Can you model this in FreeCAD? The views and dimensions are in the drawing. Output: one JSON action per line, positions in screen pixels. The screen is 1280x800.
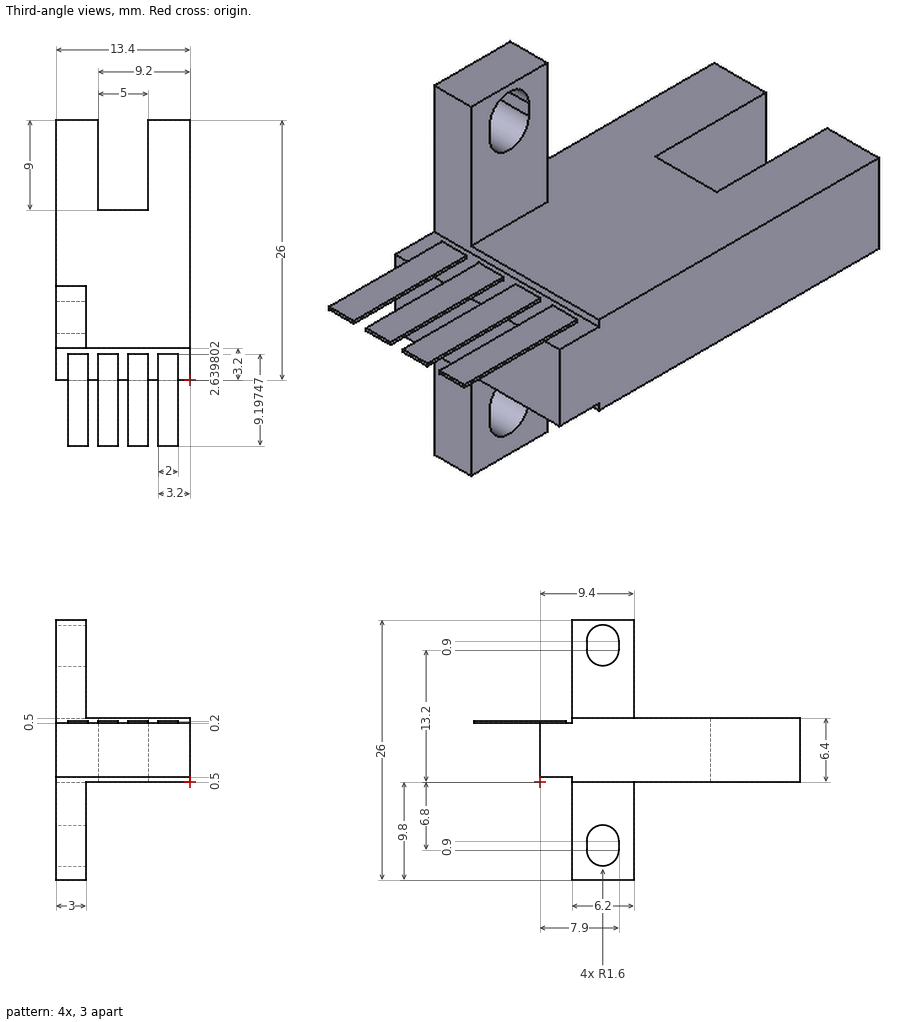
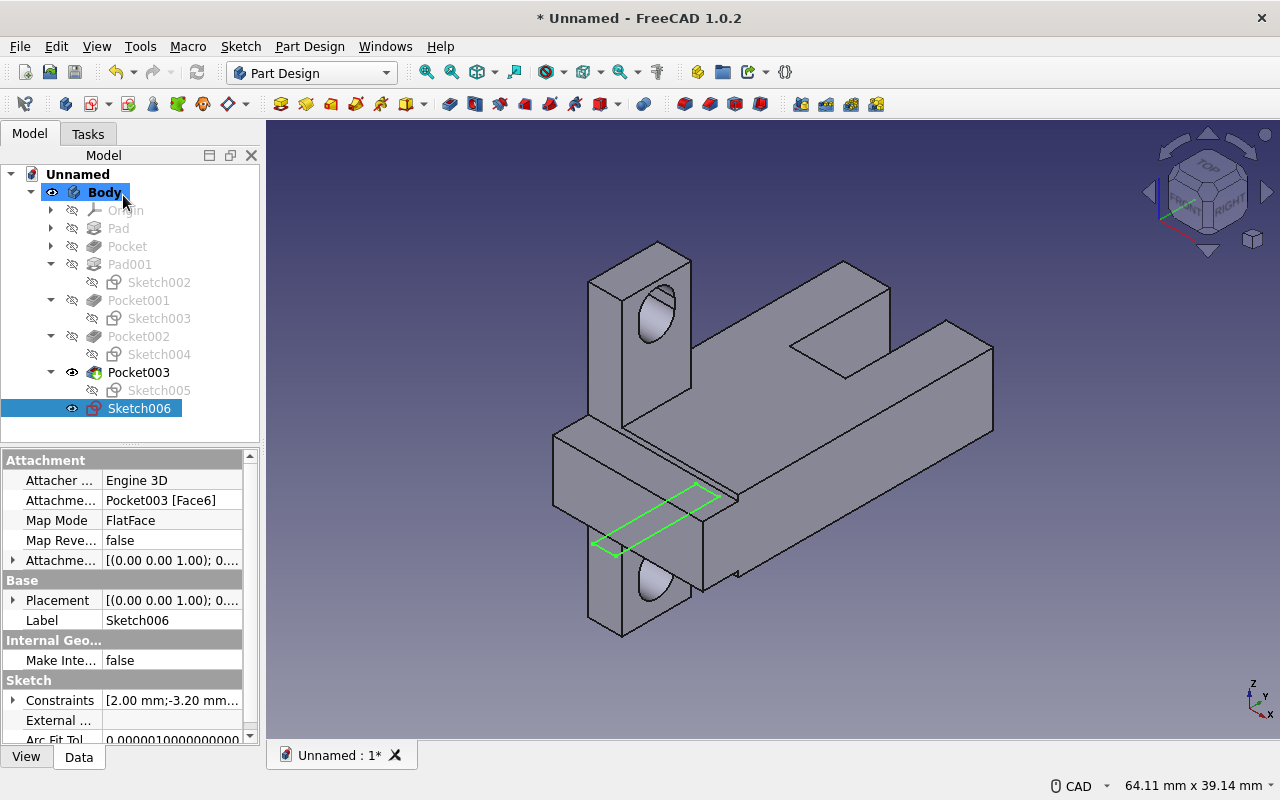
{"action": "left_click", "coordinate": [281, 104]}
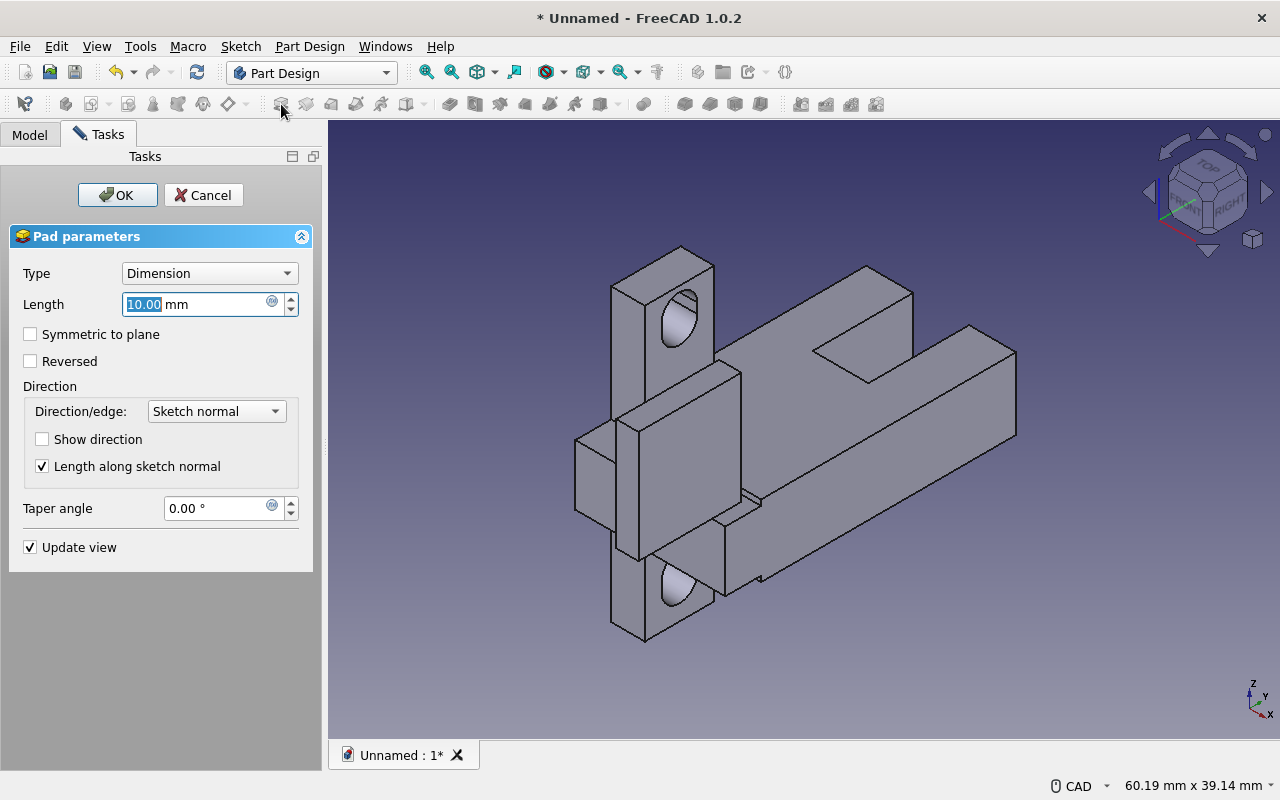
{"action": "type", "text": "0.2"}
{"action": "key", "text": "Tab"}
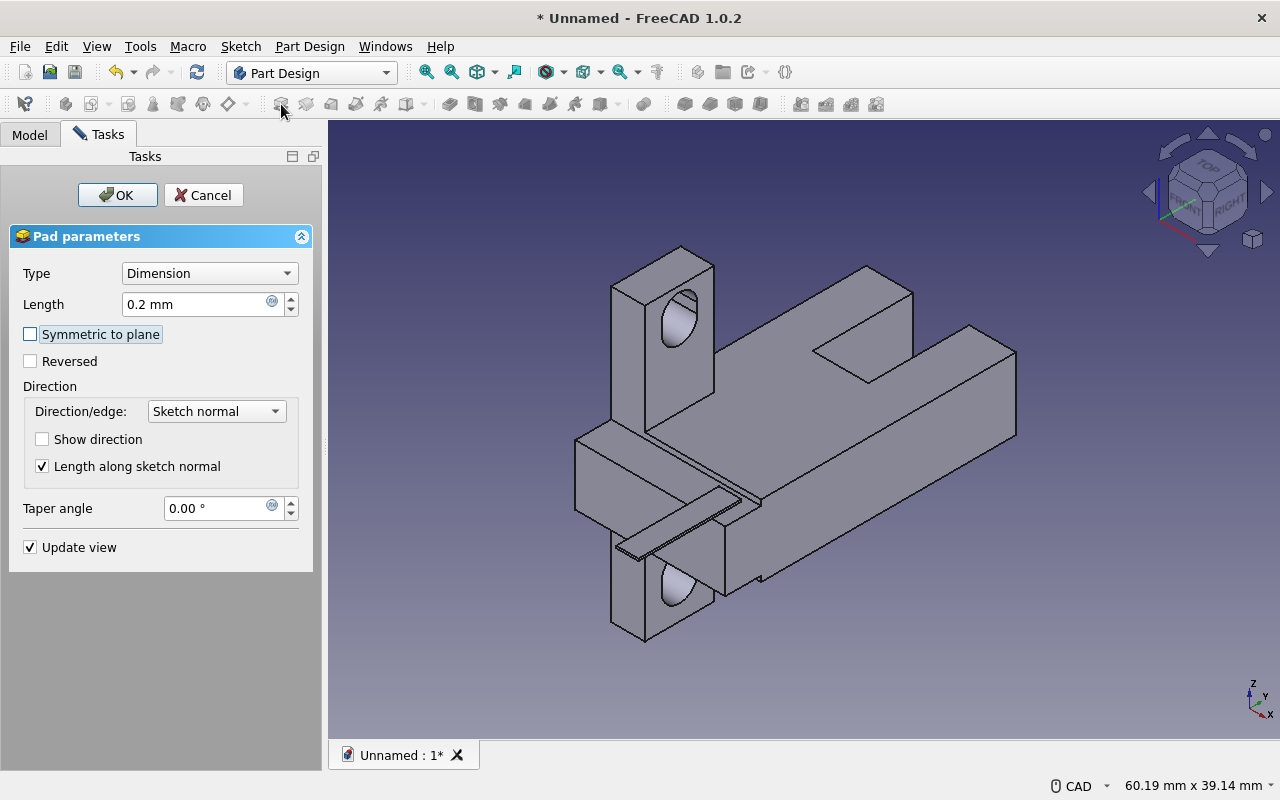
{"action": "left_click", "coordinate": [118, 195]}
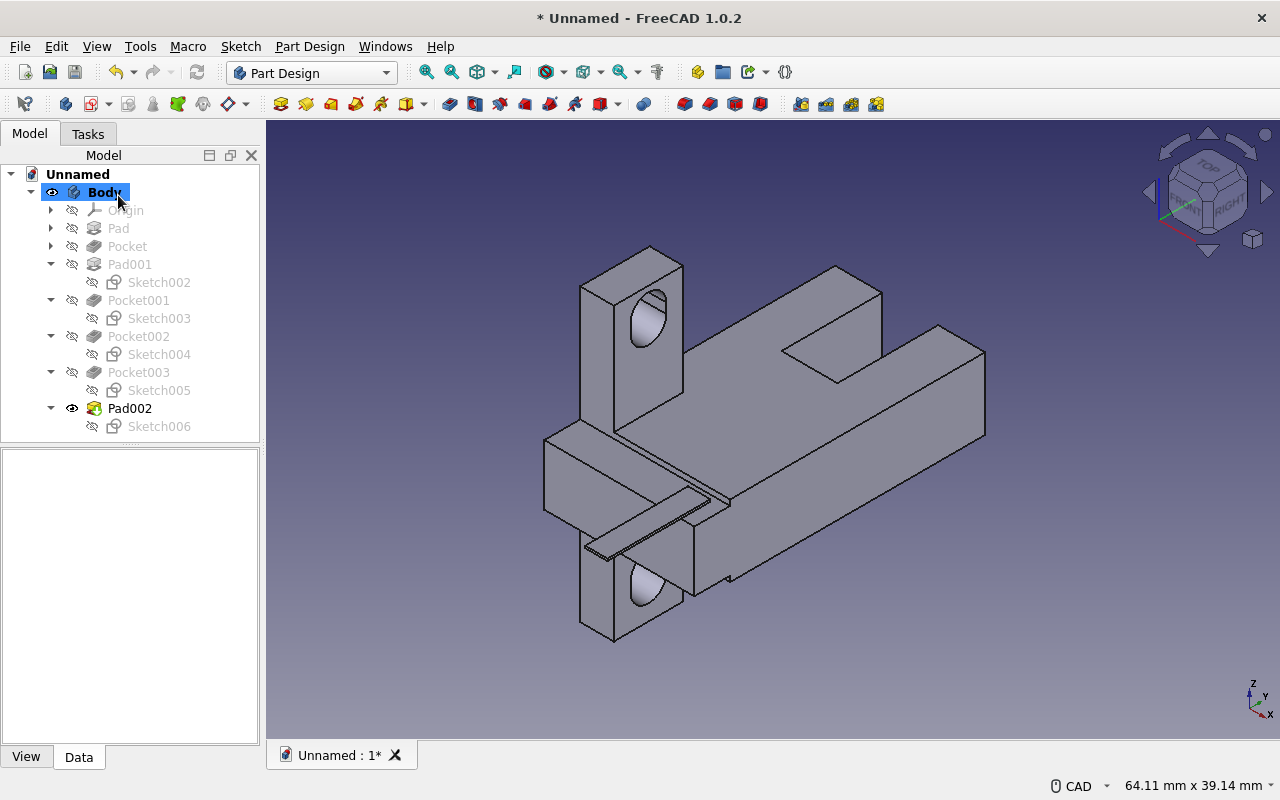
{"action": "left_click", "coordinate": [427, 72]}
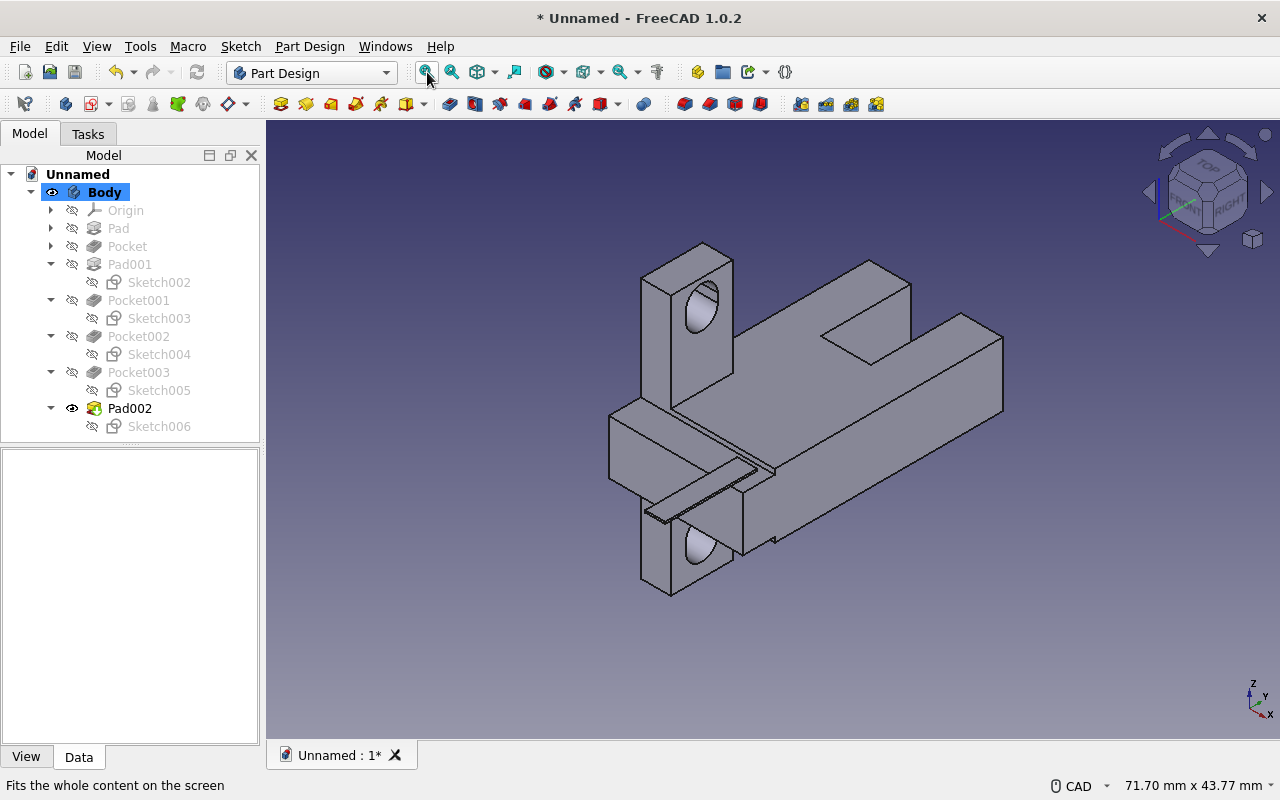
{"action": "left_click", "coordinate": [117, 408]}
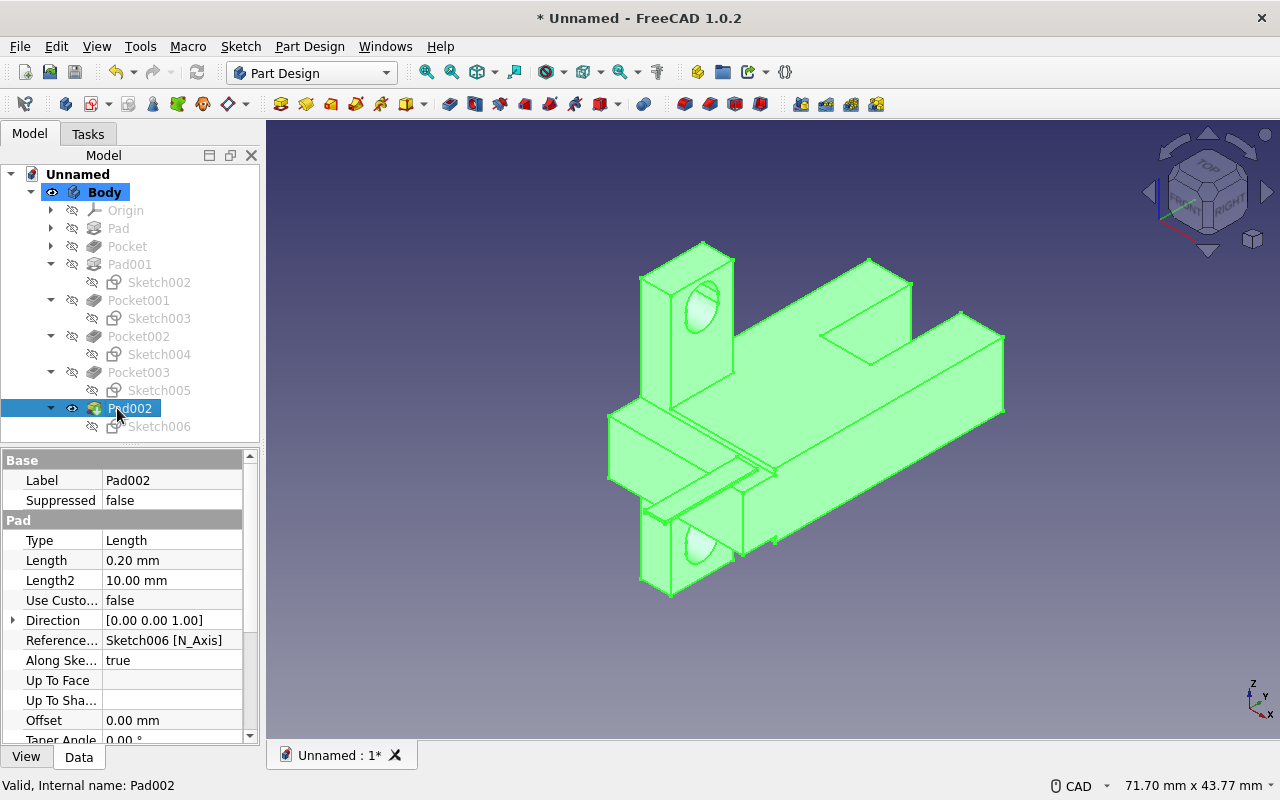
{"action": "left_click", "coordinate": [826, 104]}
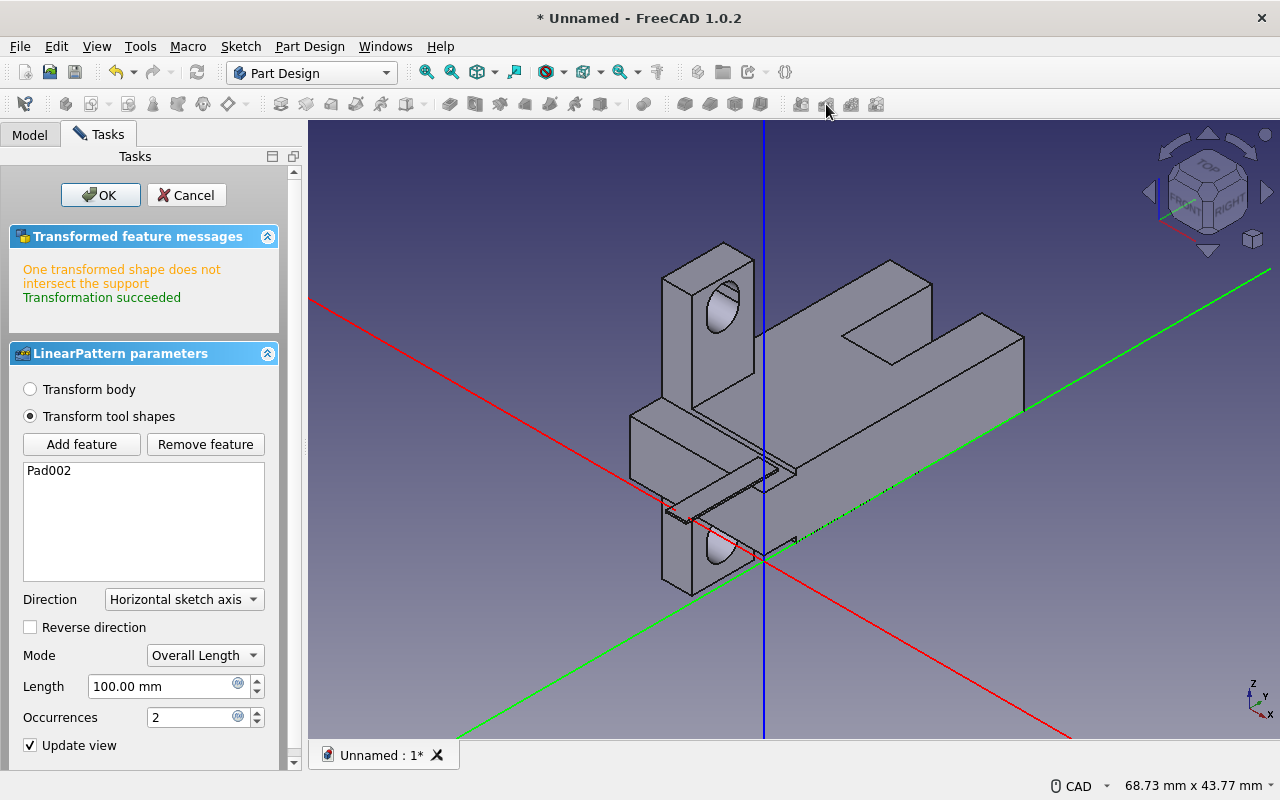
{"action": "left_click", "coordinate": [185, 600]}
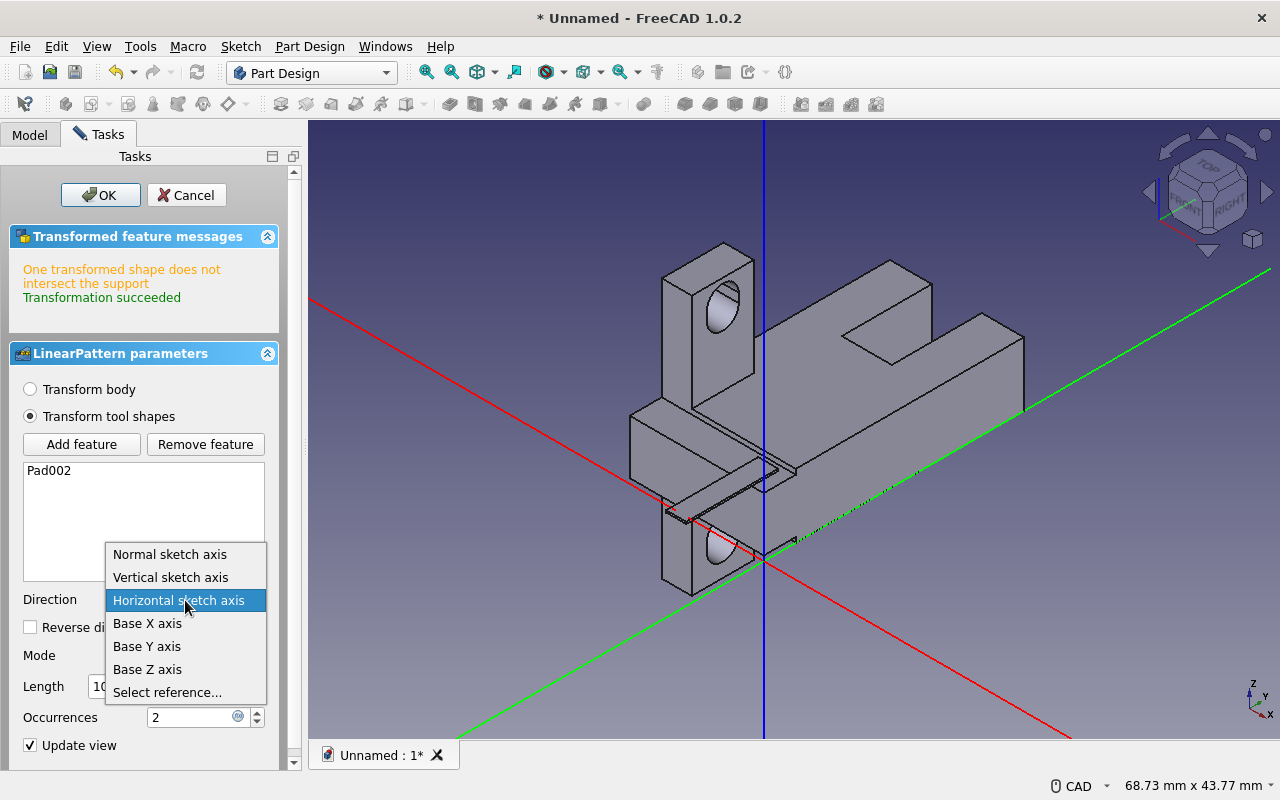
{"action": "left_click", "coordinate": [184, 624]}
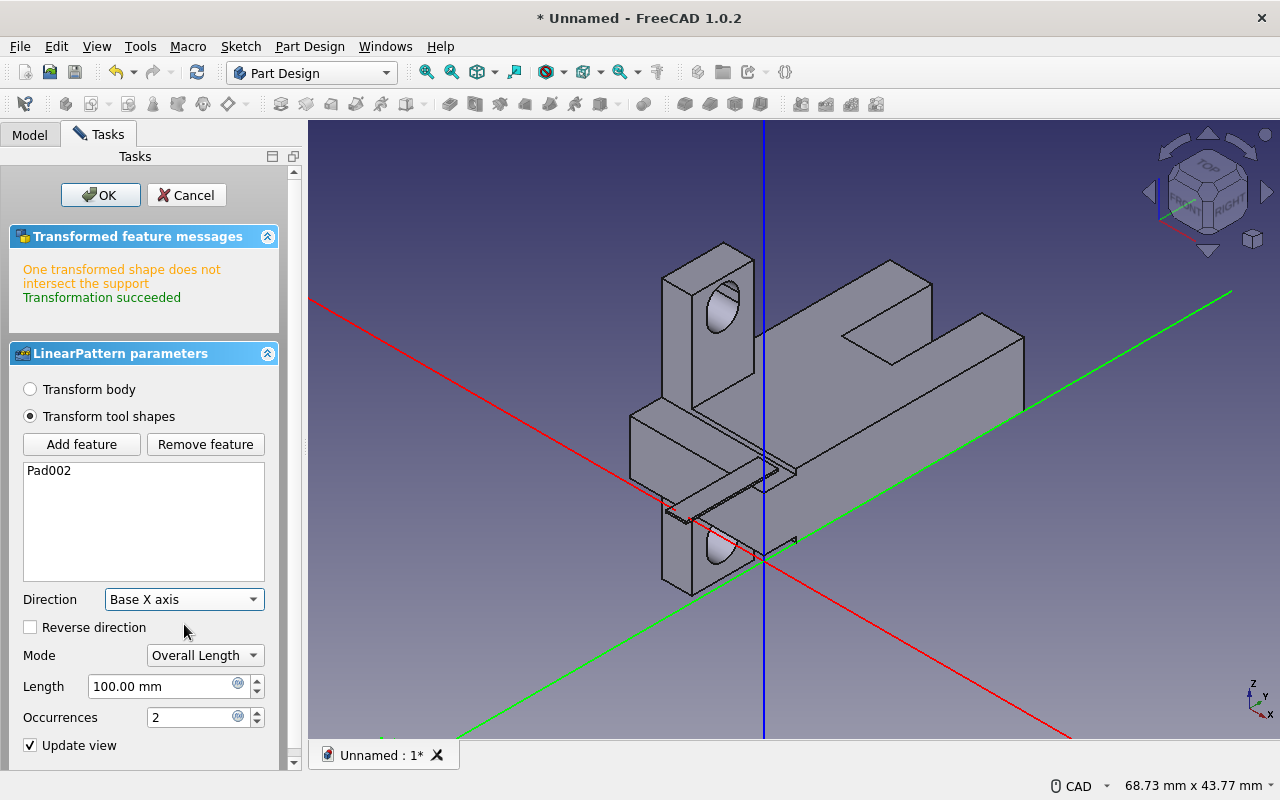
{"action": "left_click", "coordinate": [206, 656]}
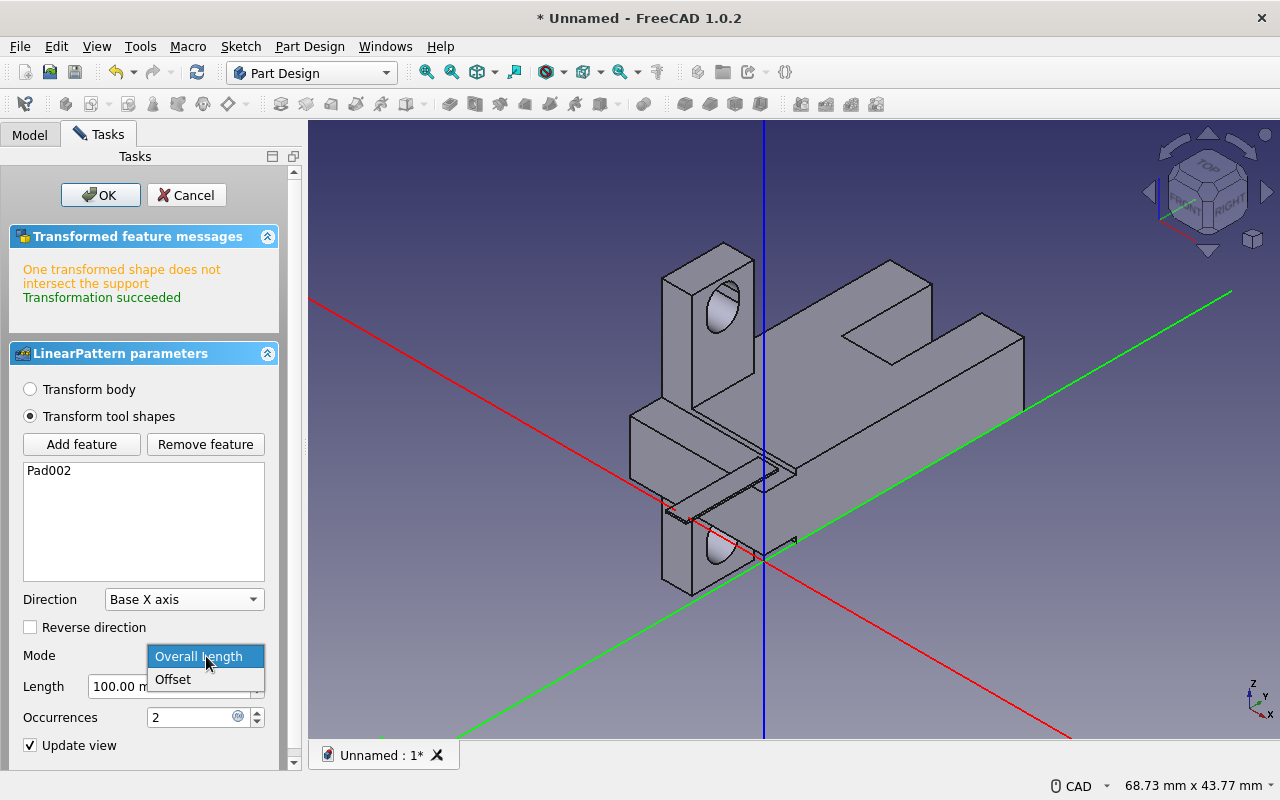
{"action": "left_click", "coordinate": [204, 680]}